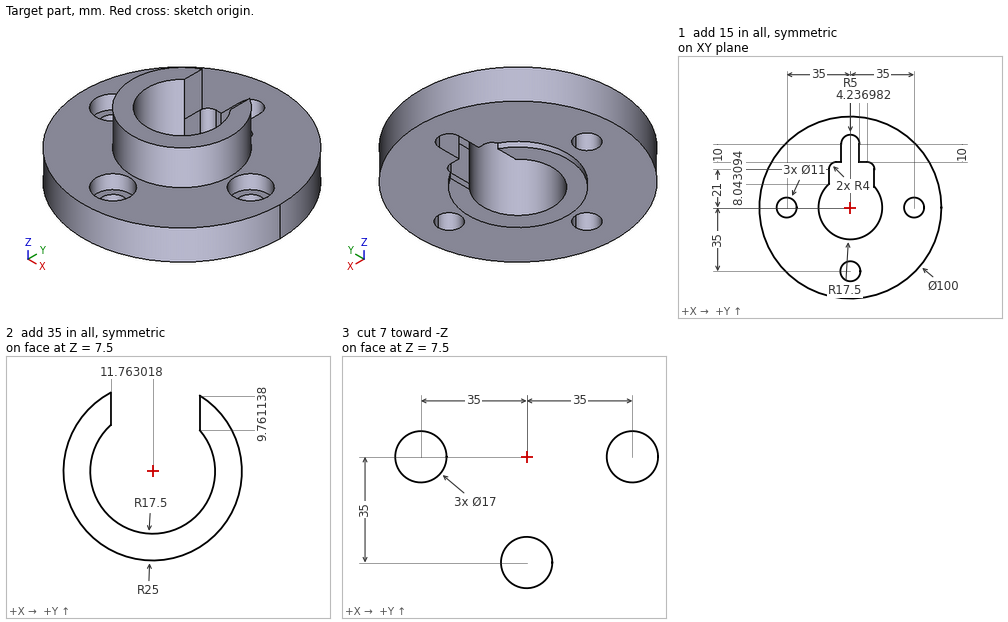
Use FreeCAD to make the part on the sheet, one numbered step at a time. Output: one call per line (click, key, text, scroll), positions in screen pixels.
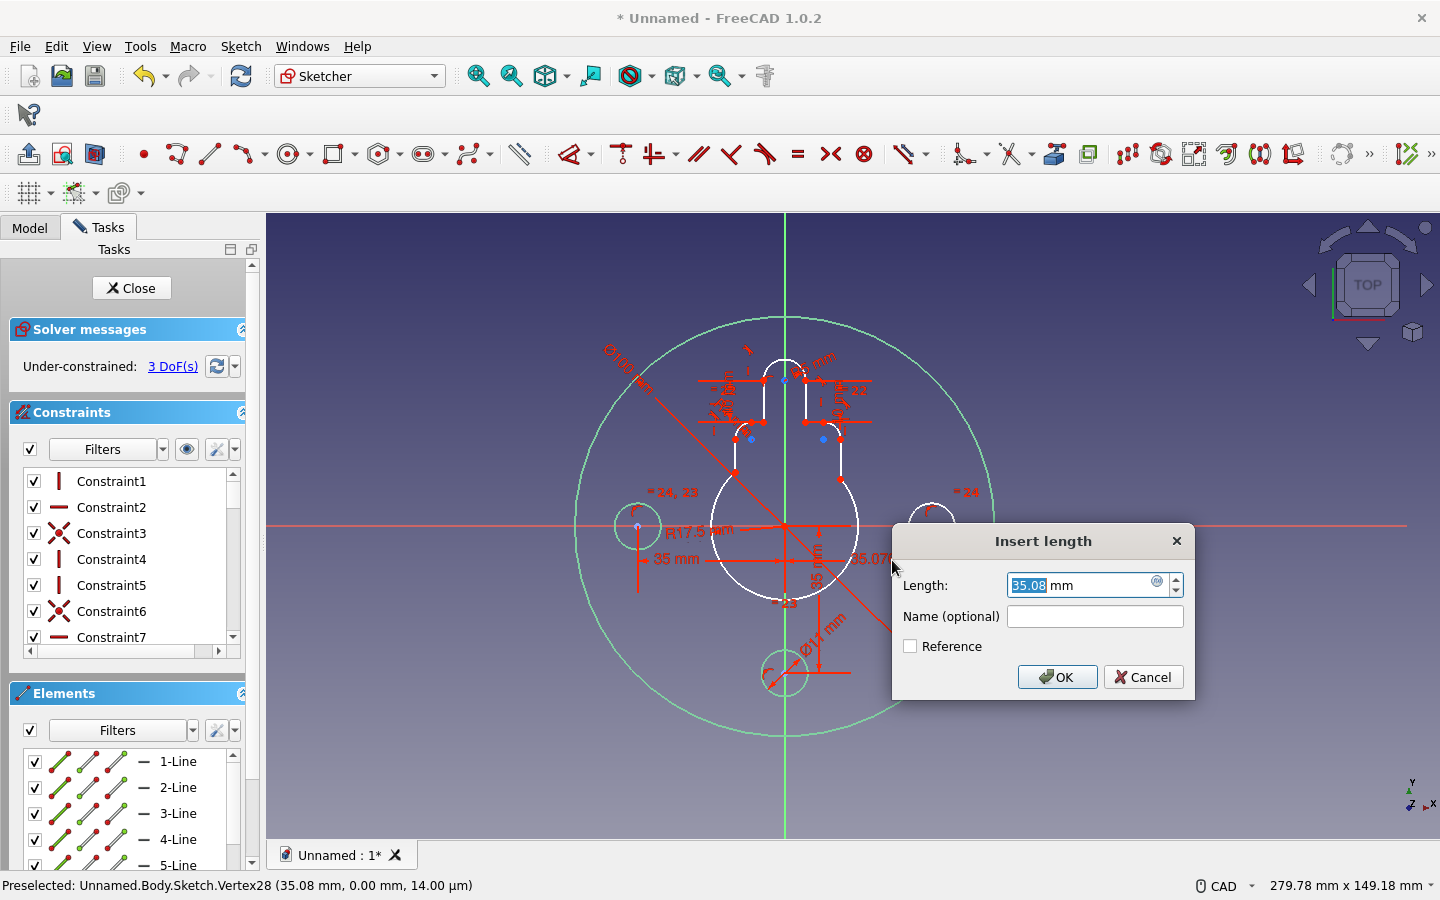
text(35)
key(Return)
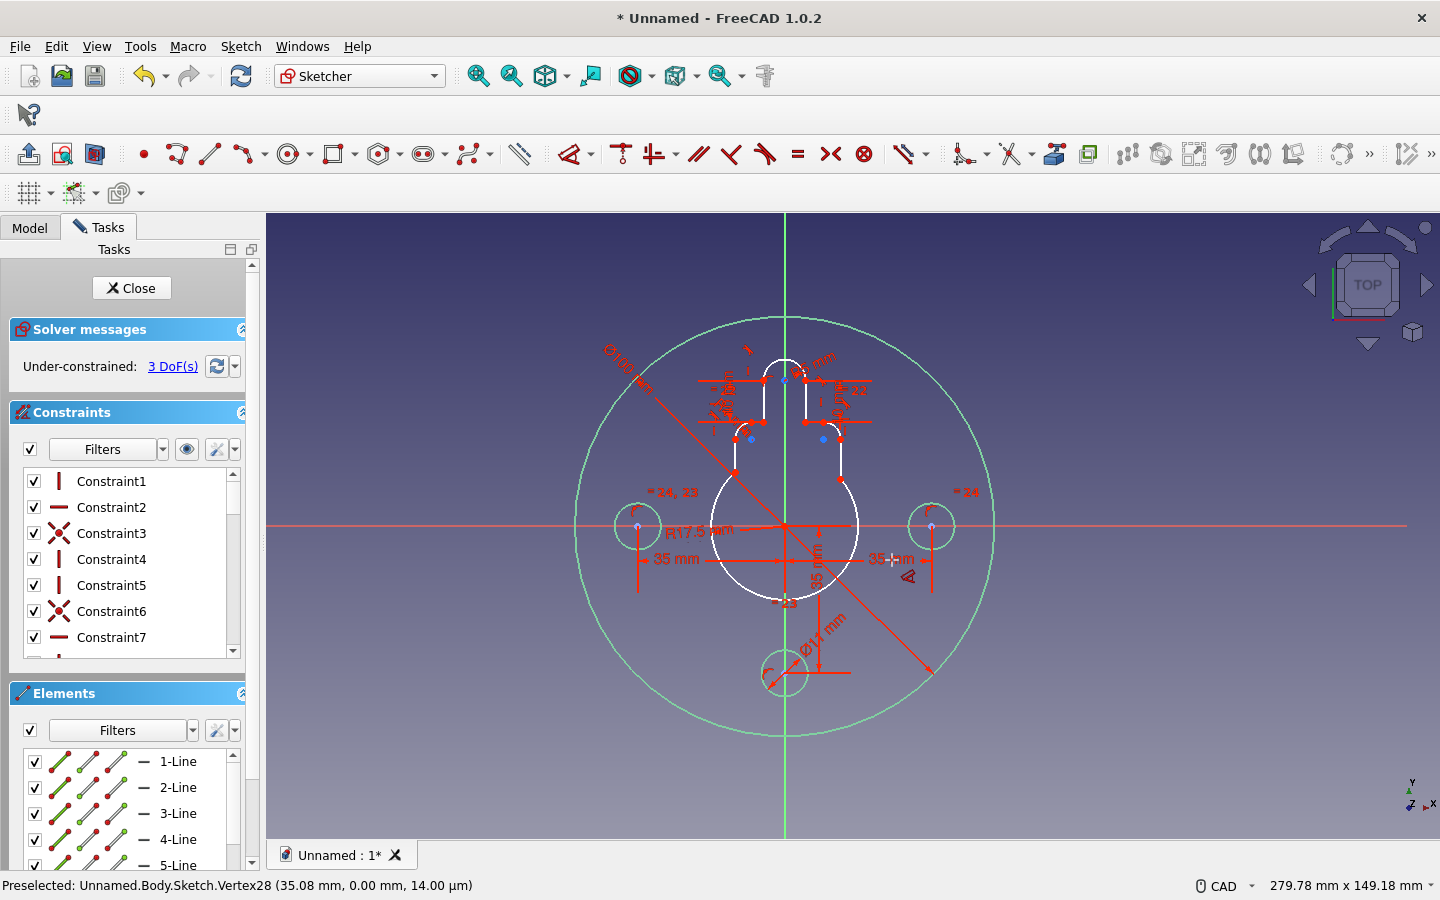
click(735, 439)
click(701, 483)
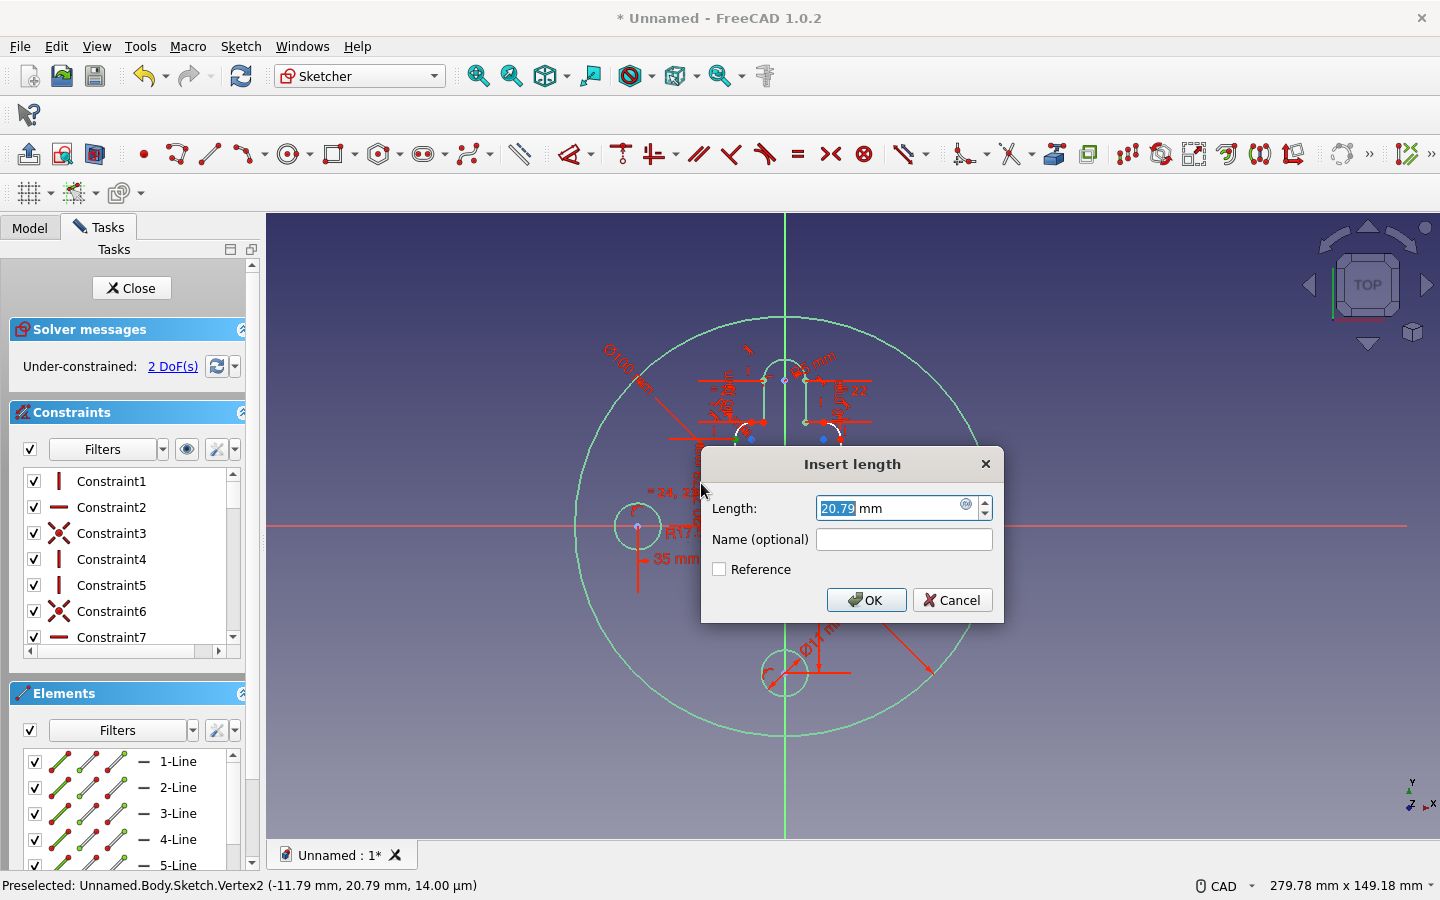
text(21)
key(Return)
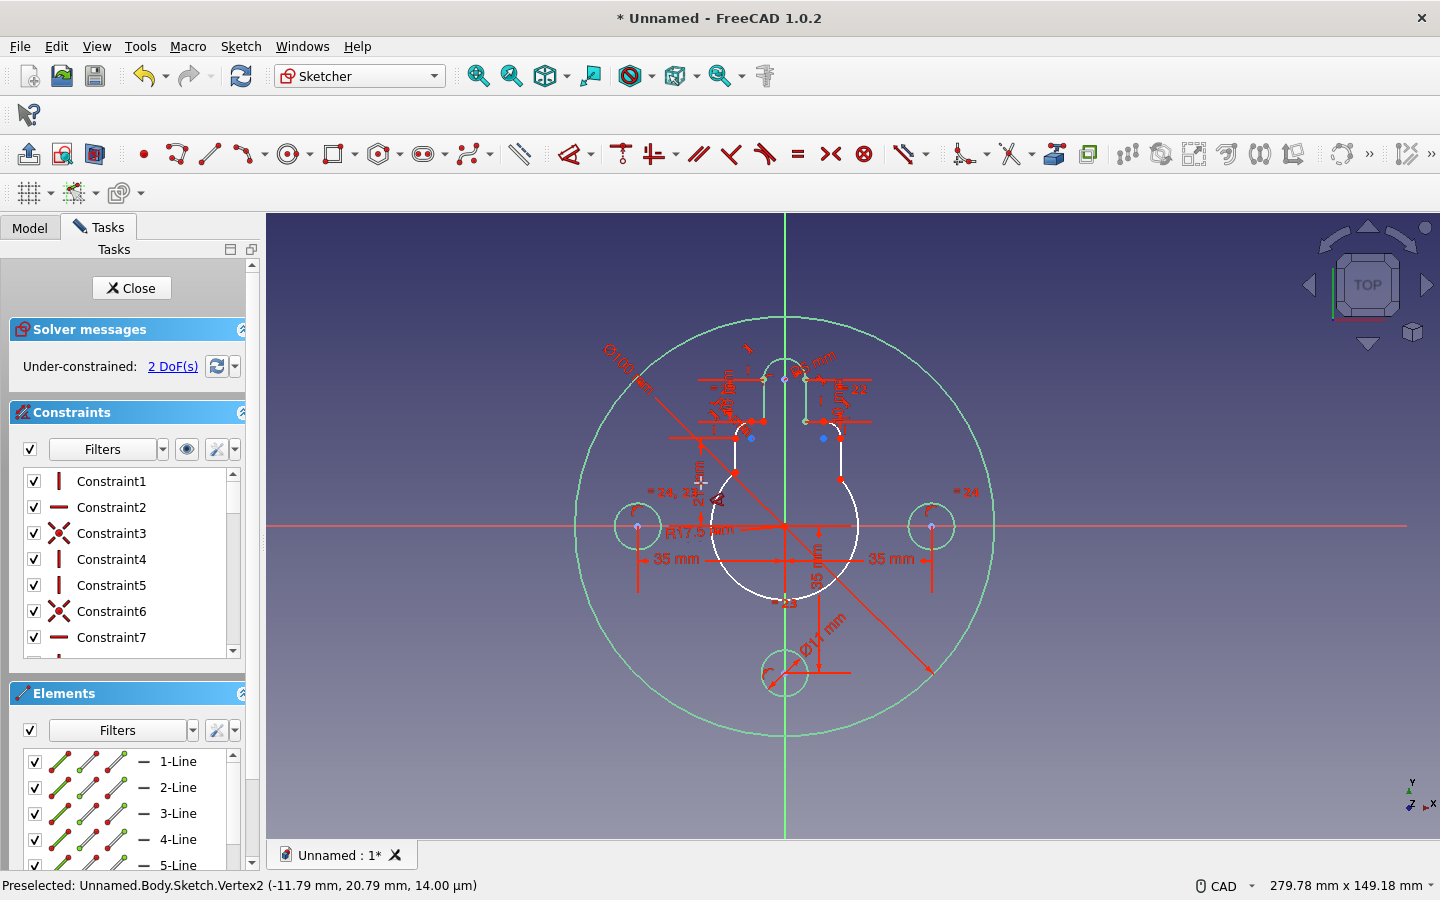
scroll(735, 462, up, 2)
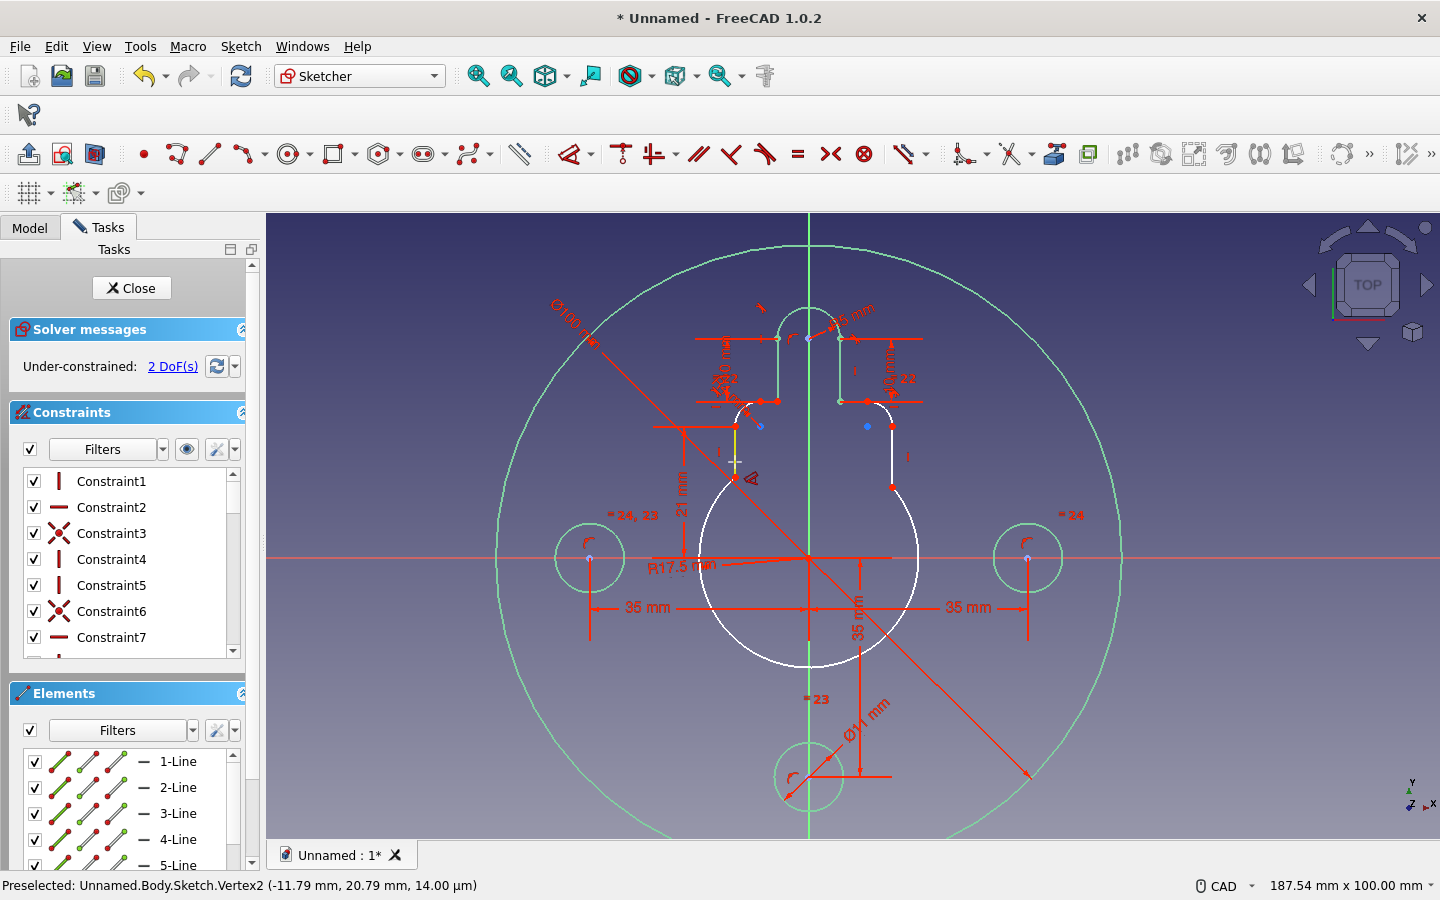
click(735, 462)
click(701, 452)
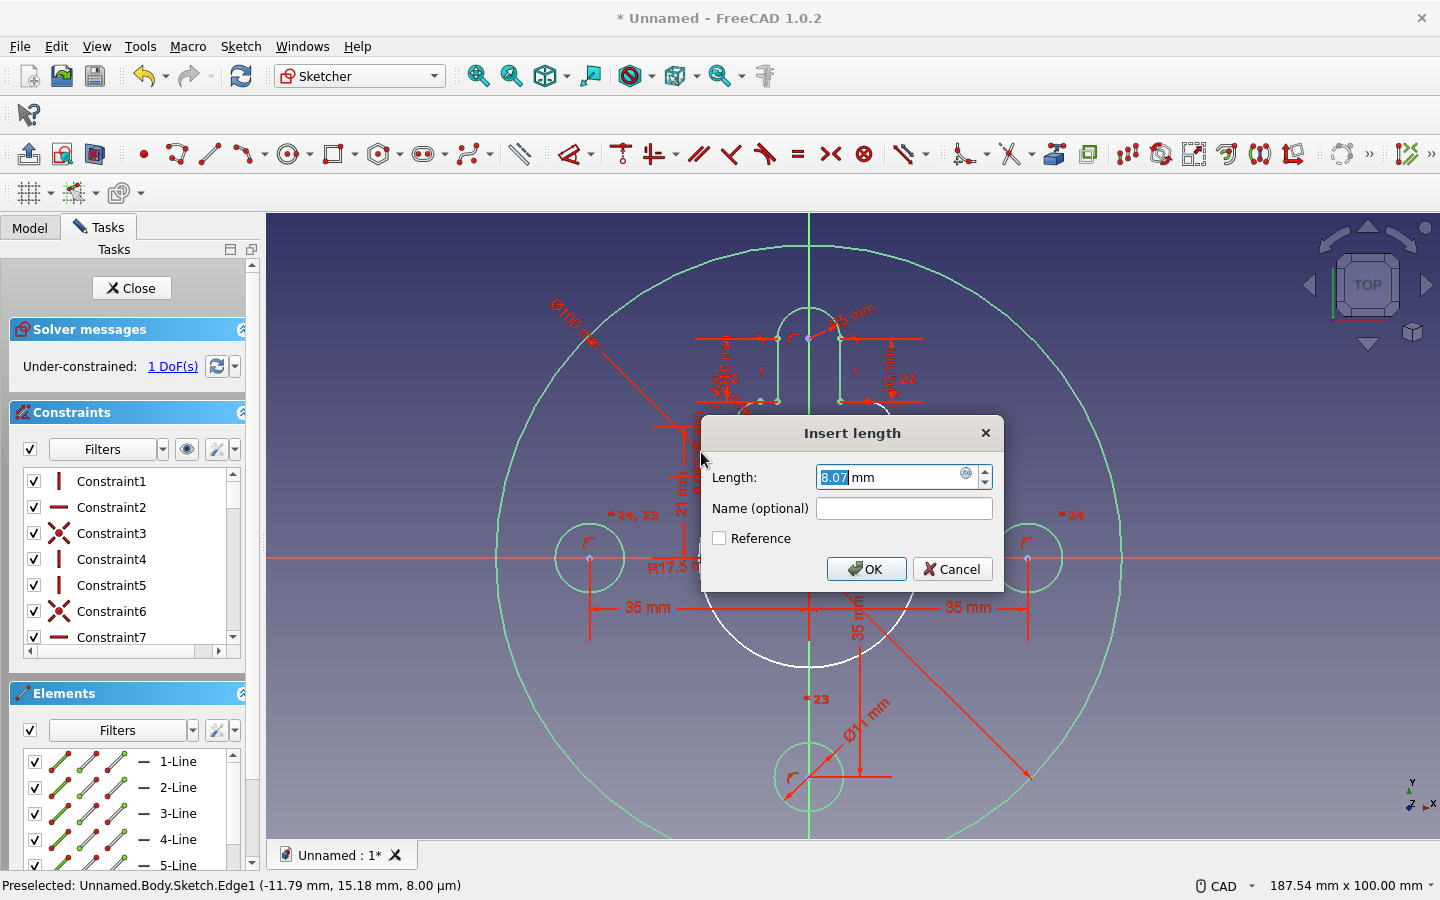
text(8.043094)
key(Return)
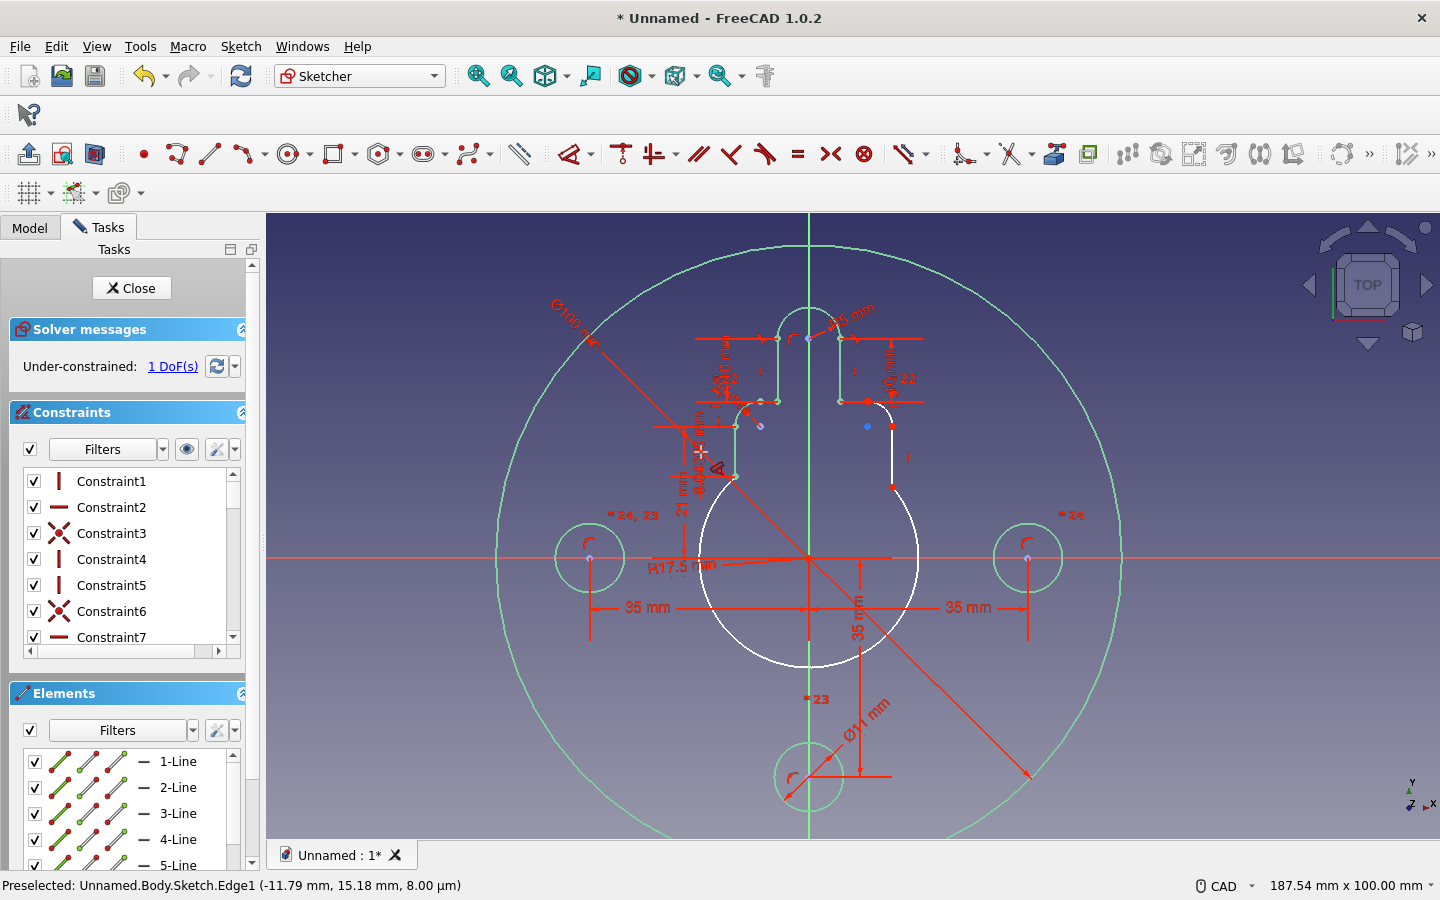
scroll(851, 402, up, 3)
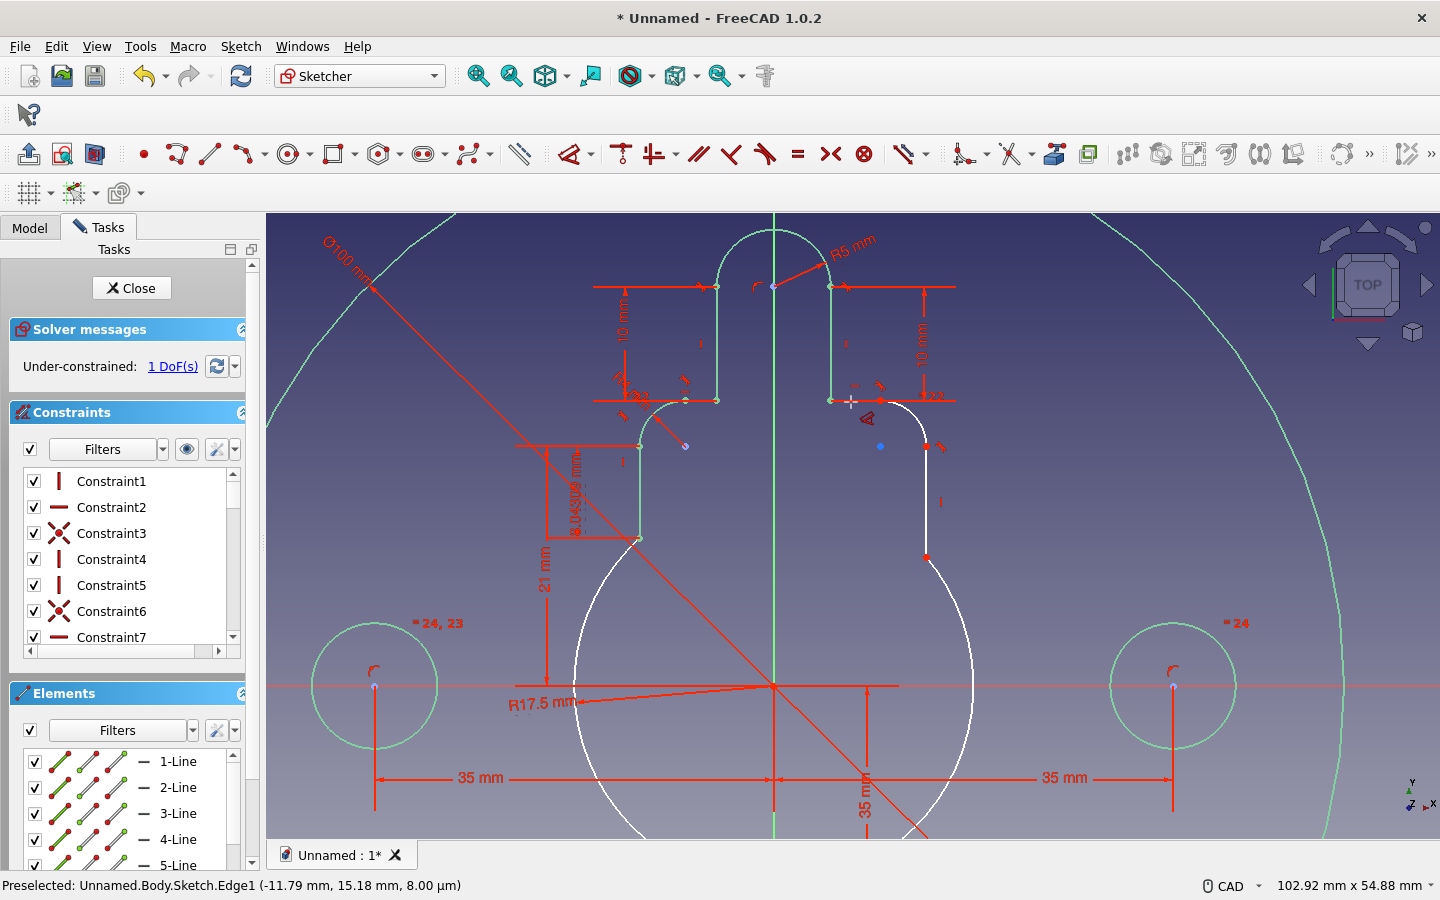
click(851, 401)
click(856, 367)